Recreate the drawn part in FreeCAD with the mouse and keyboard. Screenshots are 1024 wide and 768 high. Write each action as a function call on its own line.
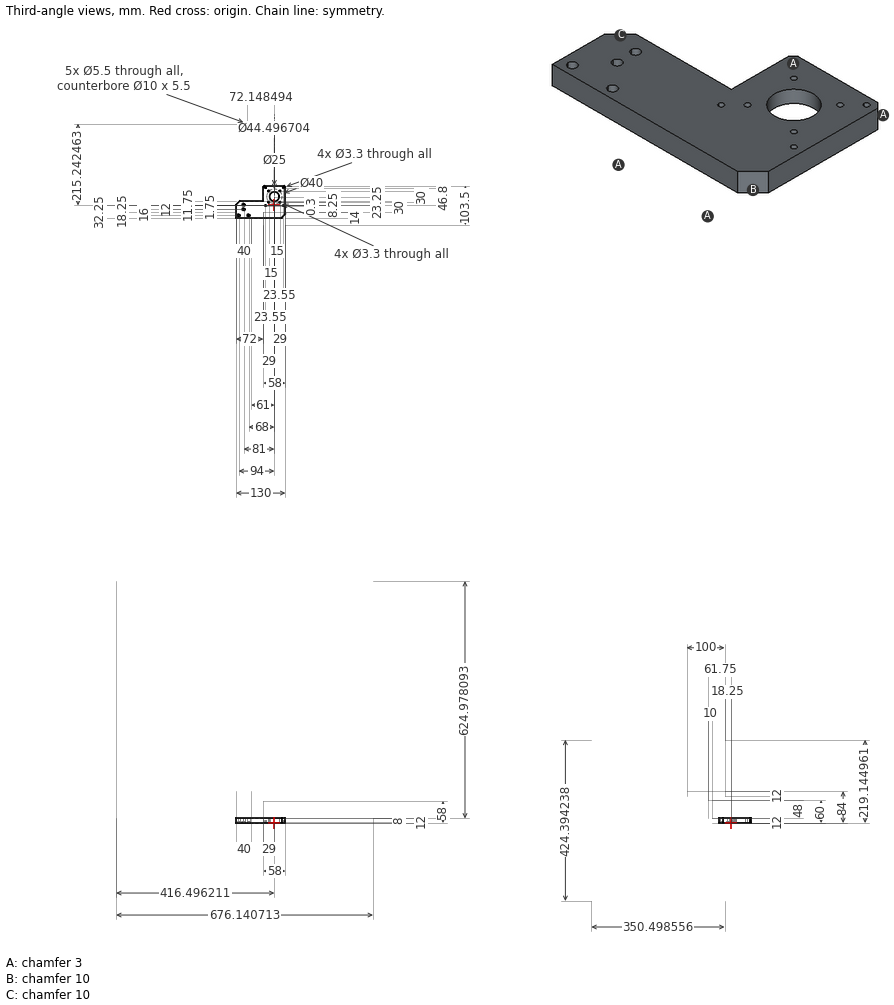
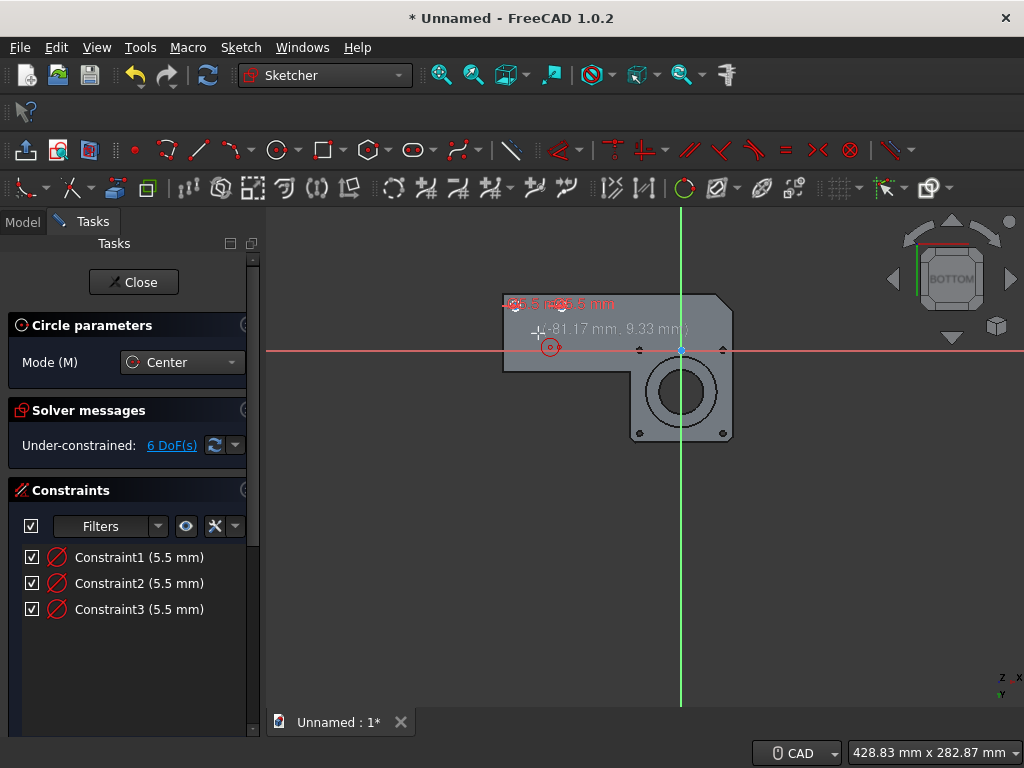
click(538, 333)
move(542, 329)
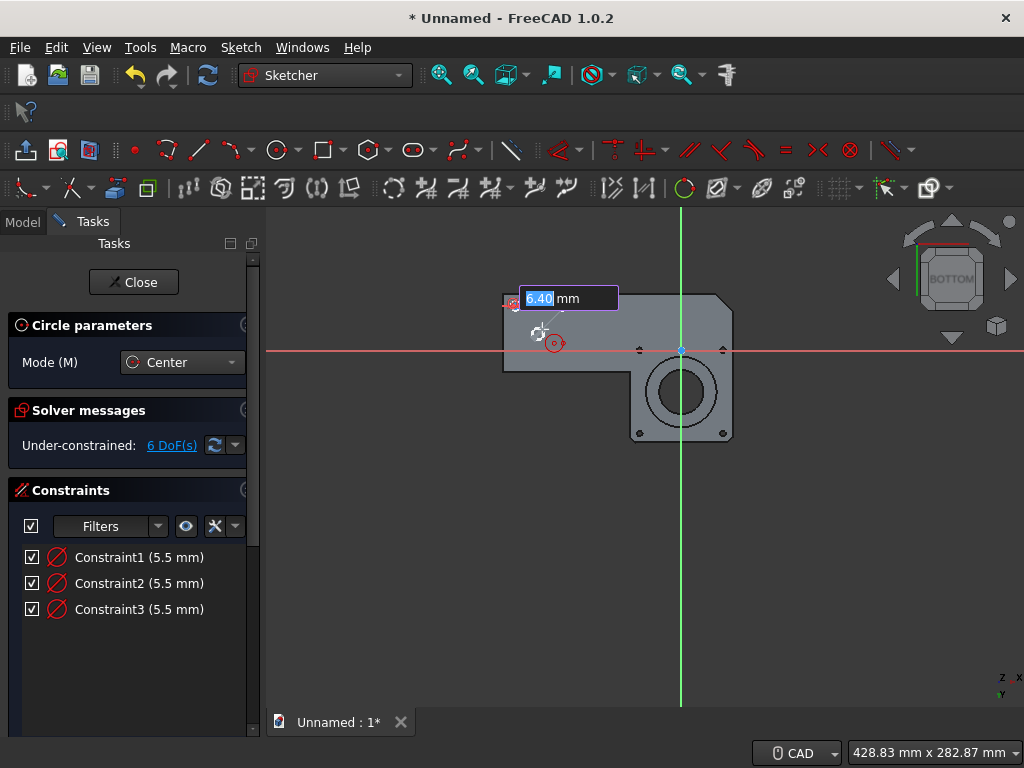
text(5.5)
key(Return)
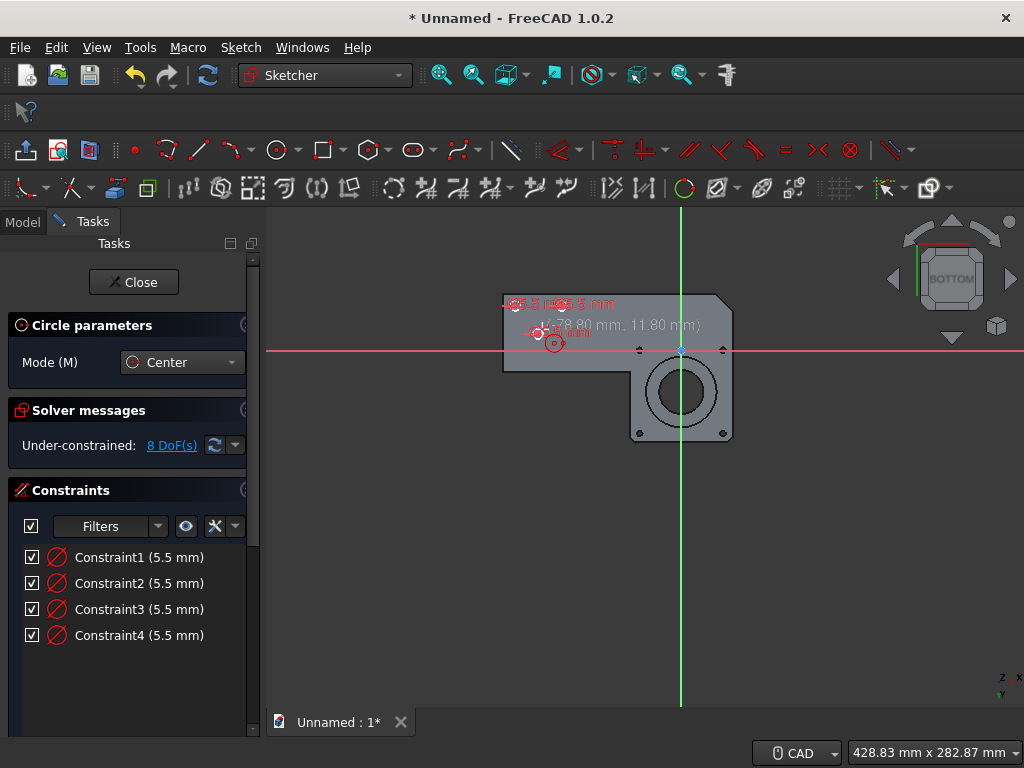
scroll(538, 354, up, 9)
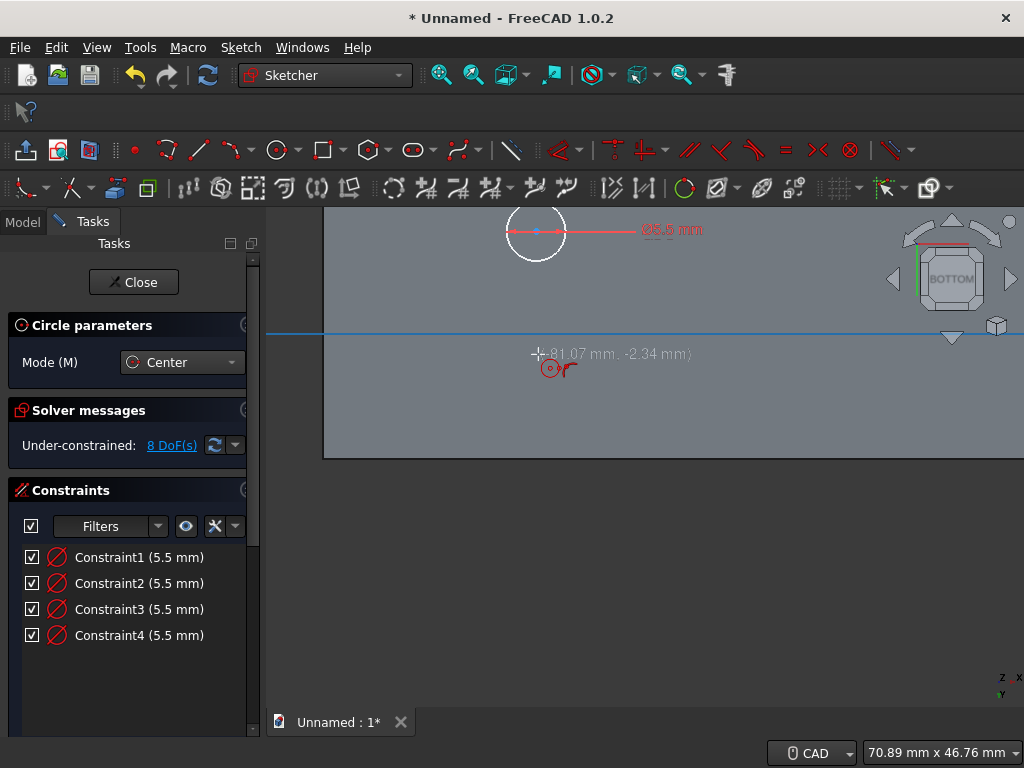
click(537, 352)
move(558, 373)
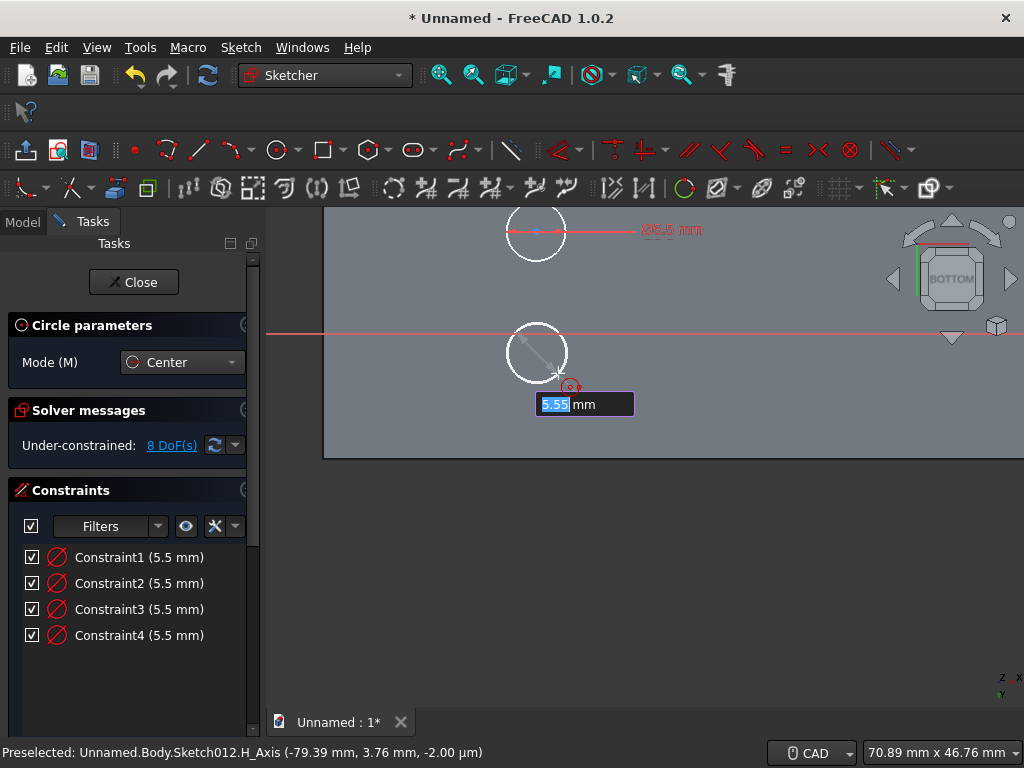
text(5.5)
key(Return)
key(Escape)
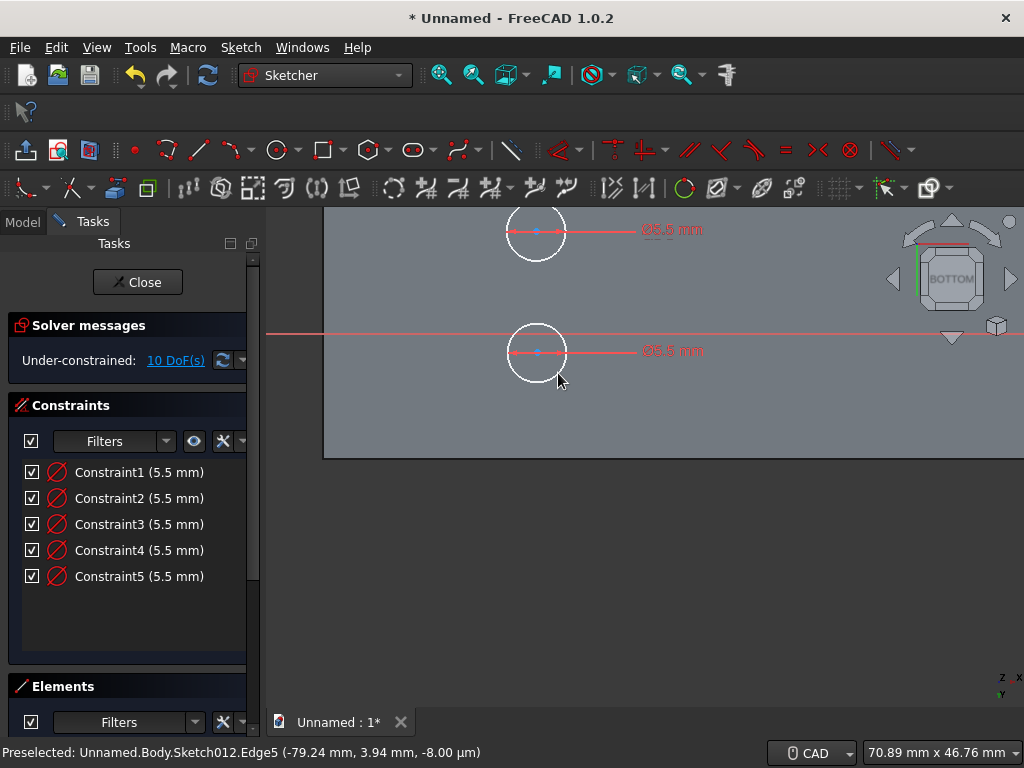
key(d)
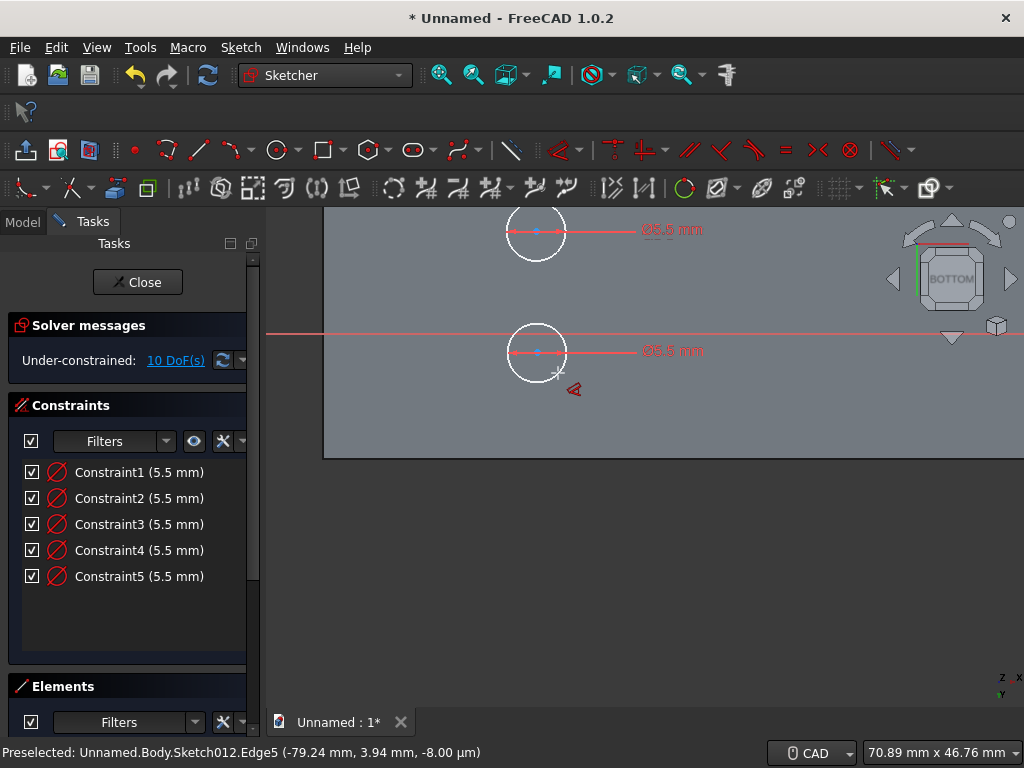
scroll(538, 346, down, 11)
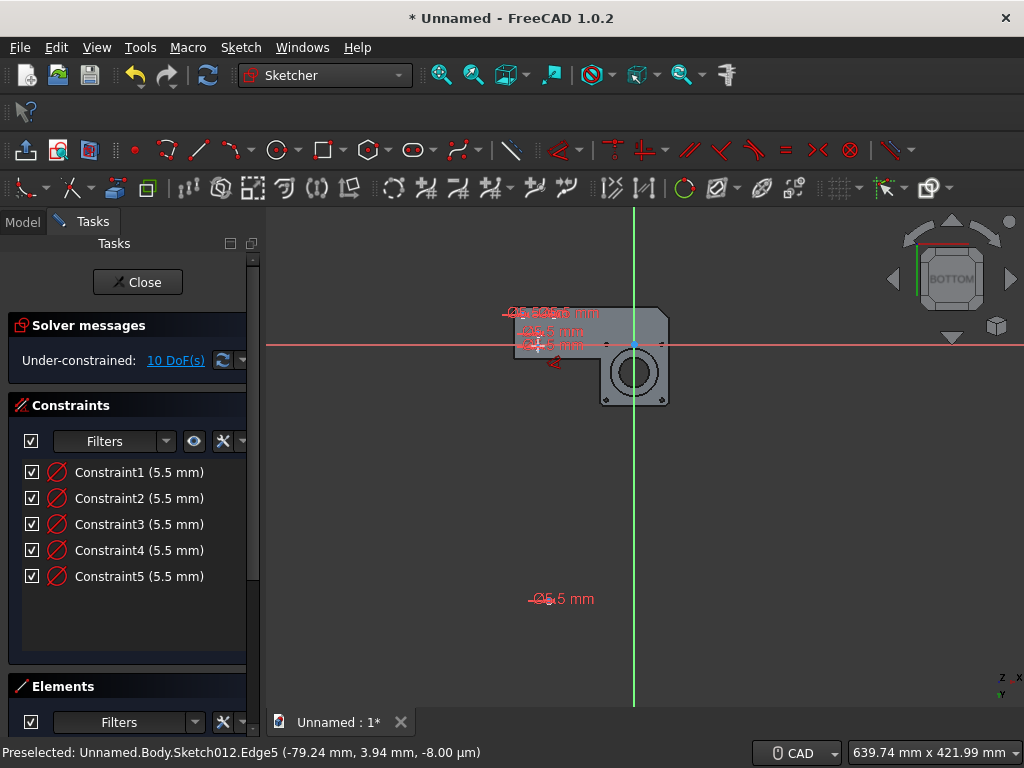
click(523, 315)
click(579, 281)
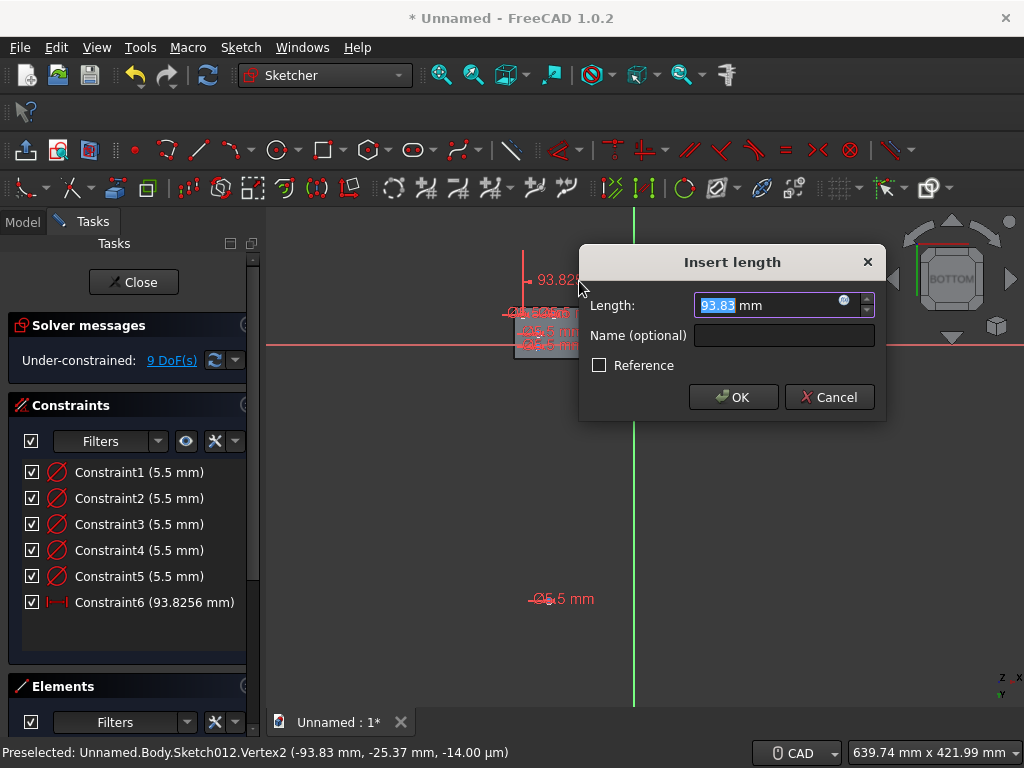
text(94)
key(Return)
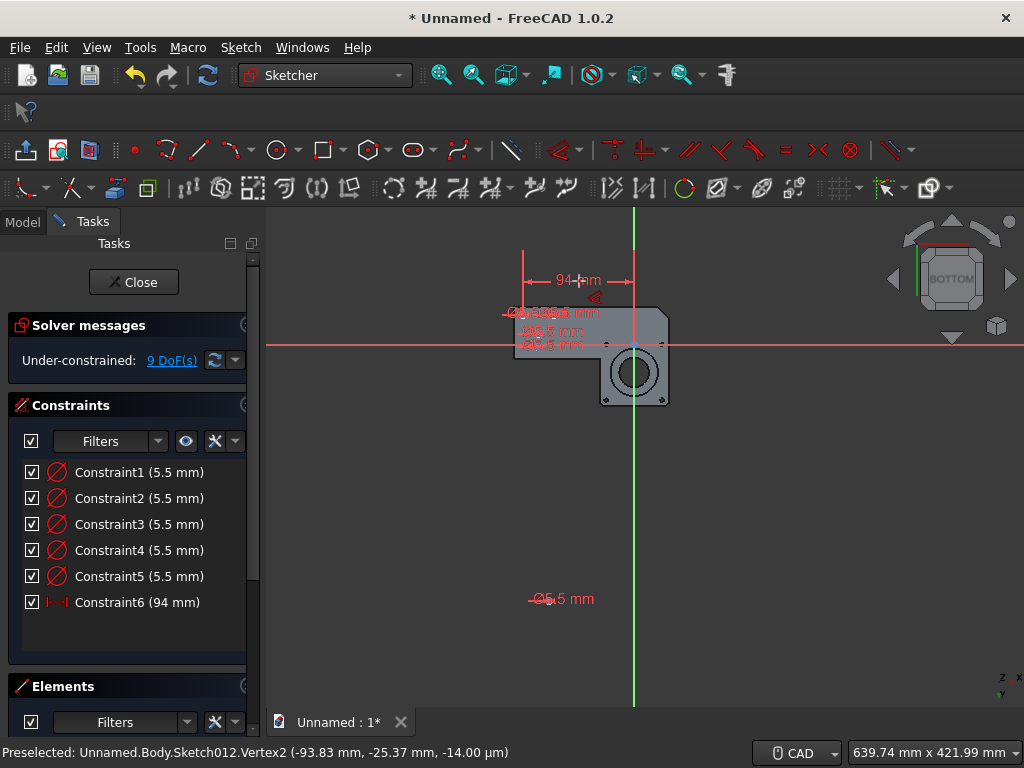
click(554, 315)
click(594, 379)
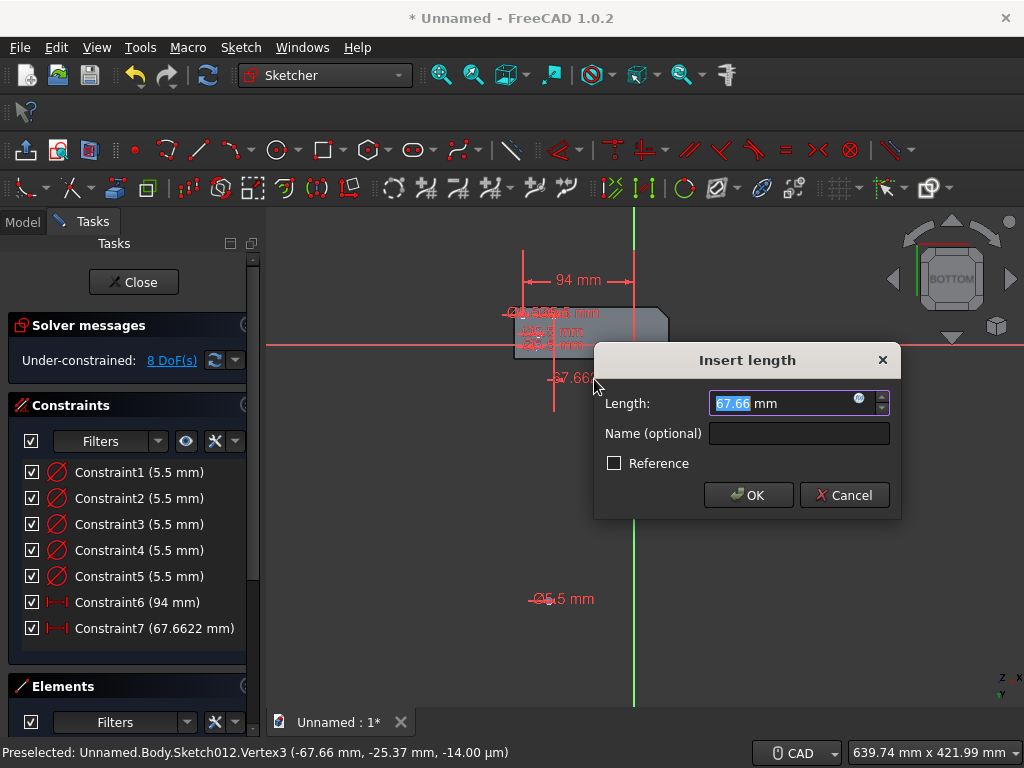
text(68)
key(Return)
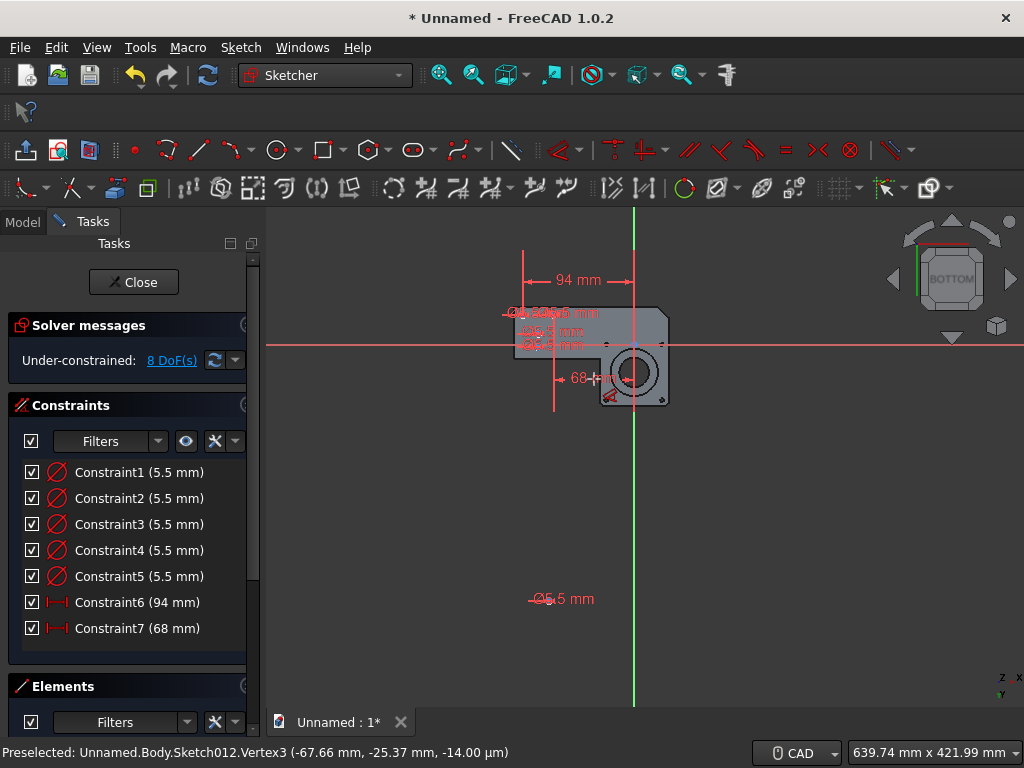
click(538, 334)
click(586, 403)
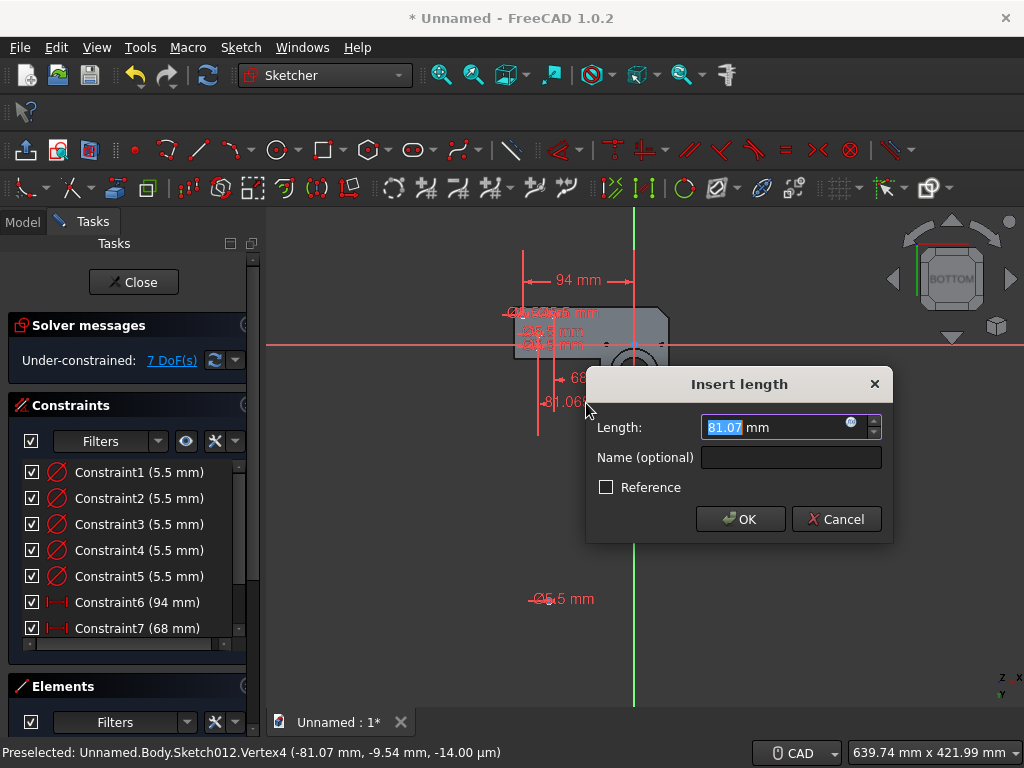
text(81)
key(Return)